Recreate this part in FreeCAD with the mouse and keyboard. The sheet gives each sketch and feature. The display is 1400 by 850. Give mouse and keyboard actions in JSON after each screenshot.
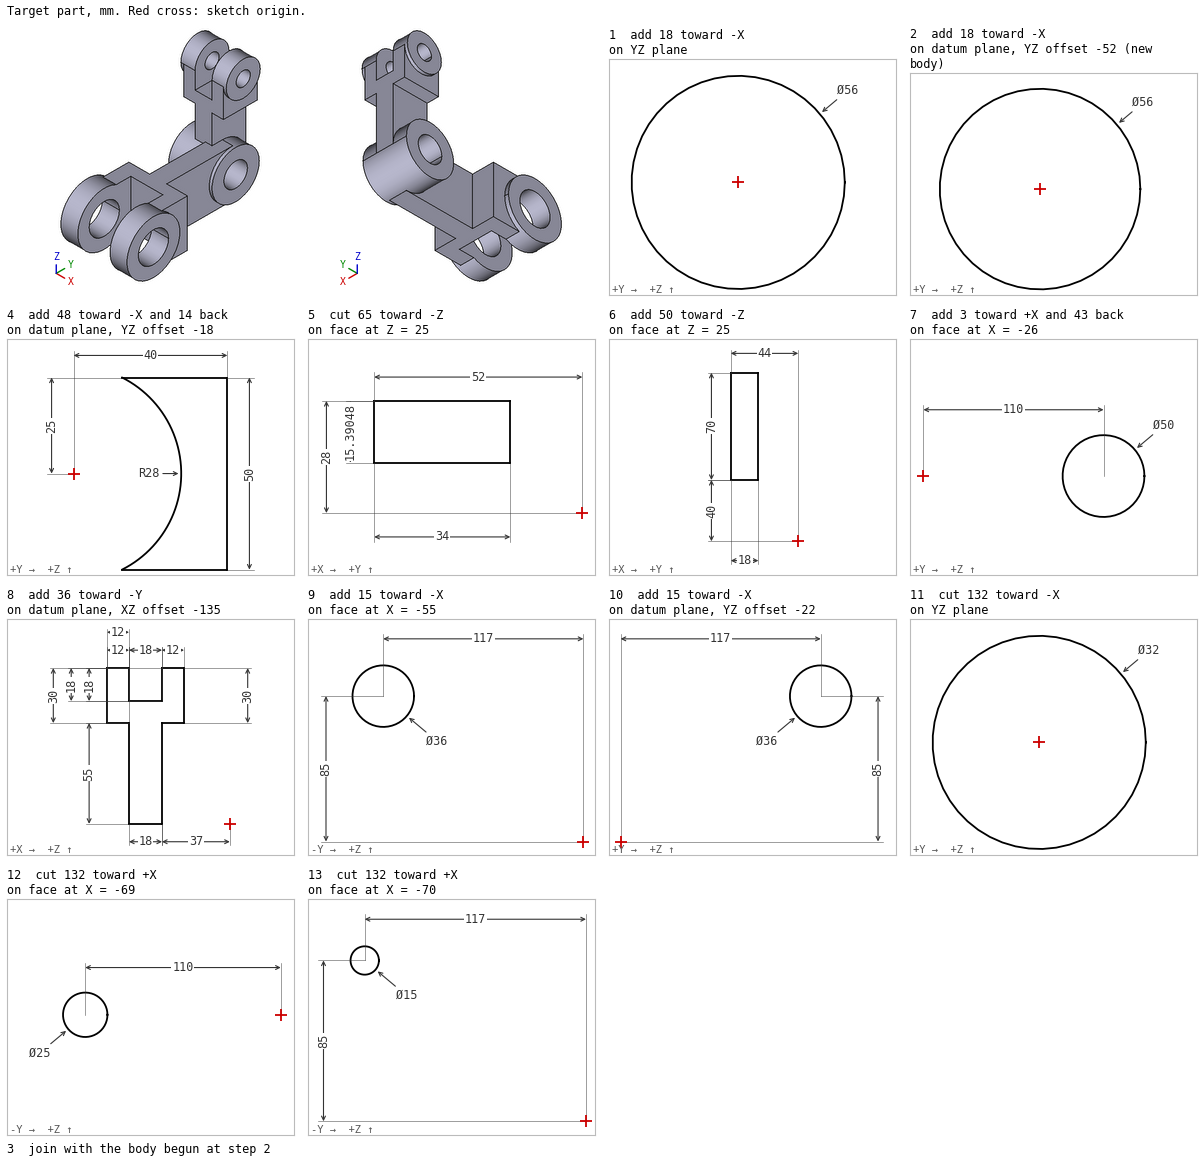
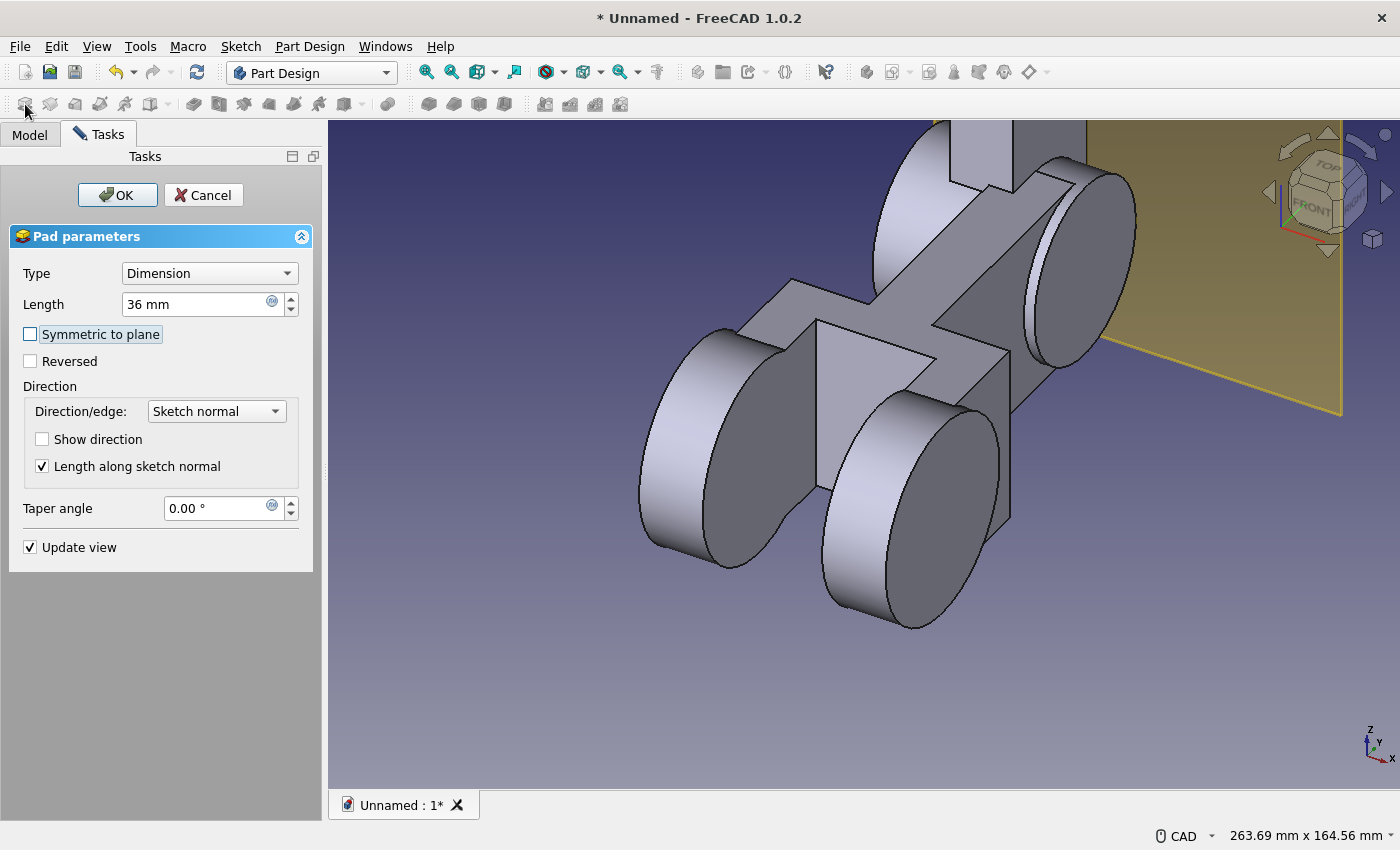
{"action": "left_click", "coordinate": [118, 195]}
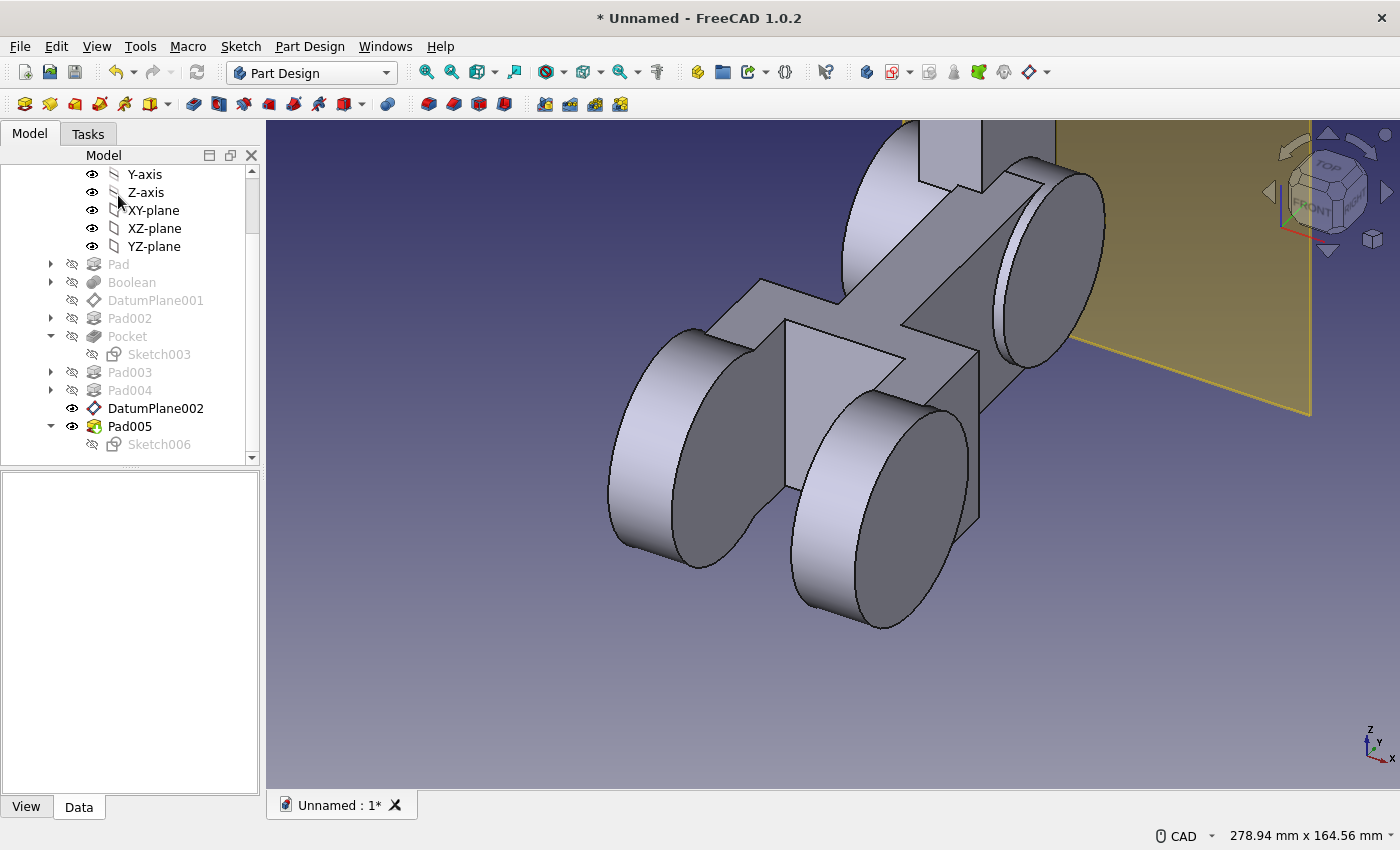
{"action": "left_click", "coordinate": [117, 408]}
{"action": "key", "text": "space"}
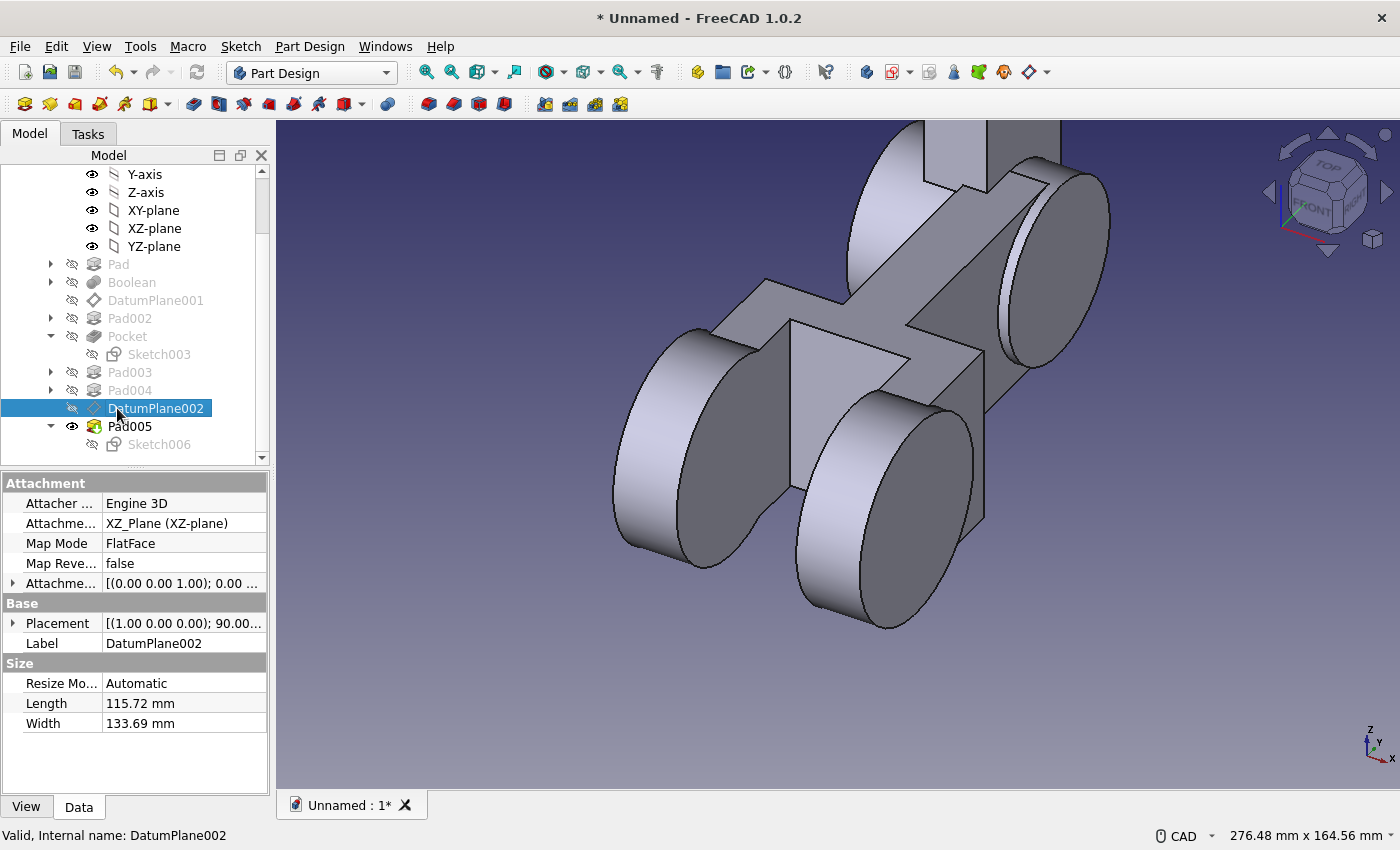
{"action": "left_click", "coordinate": [427, 72]}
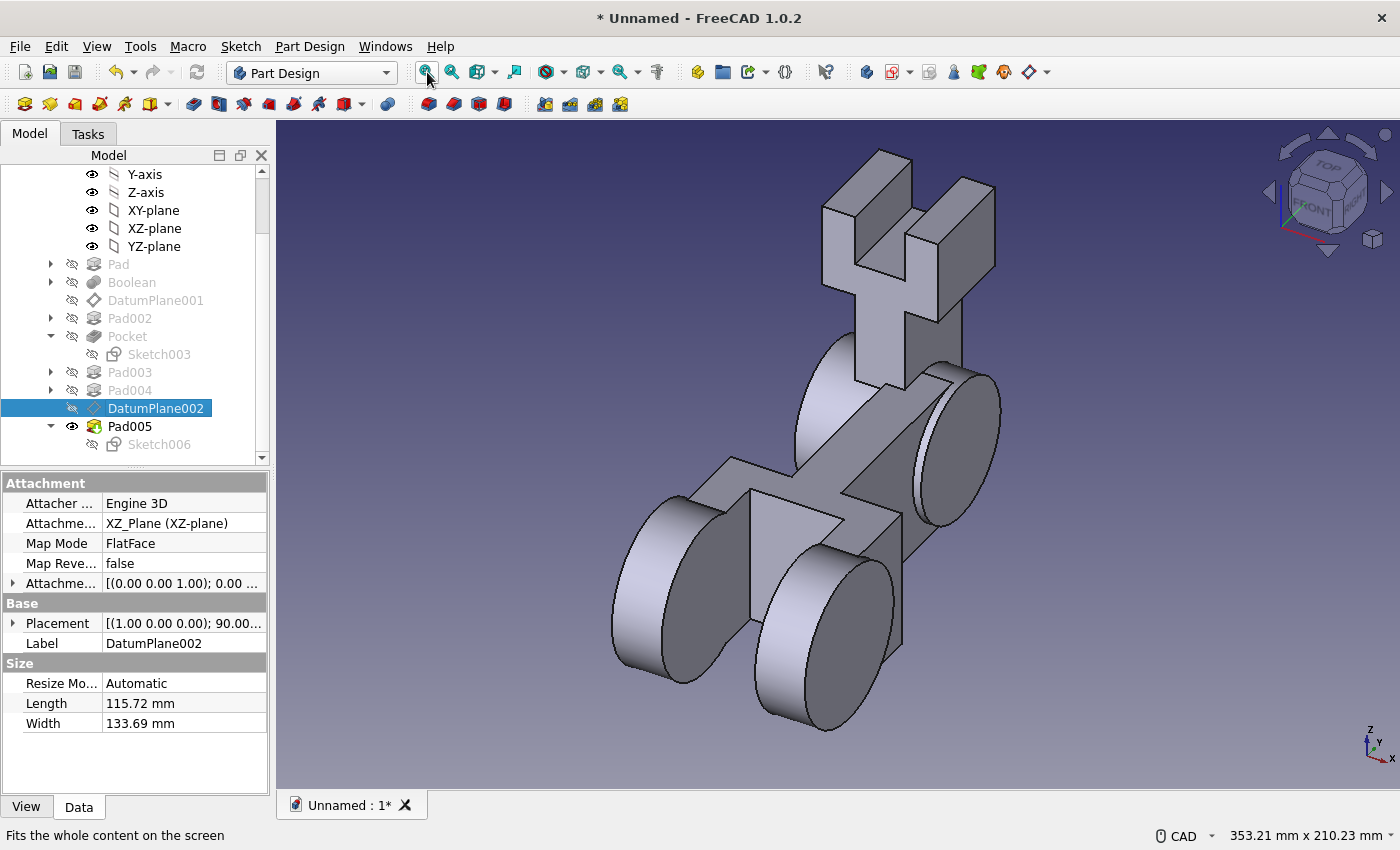
{"action": "key", "text": "6"}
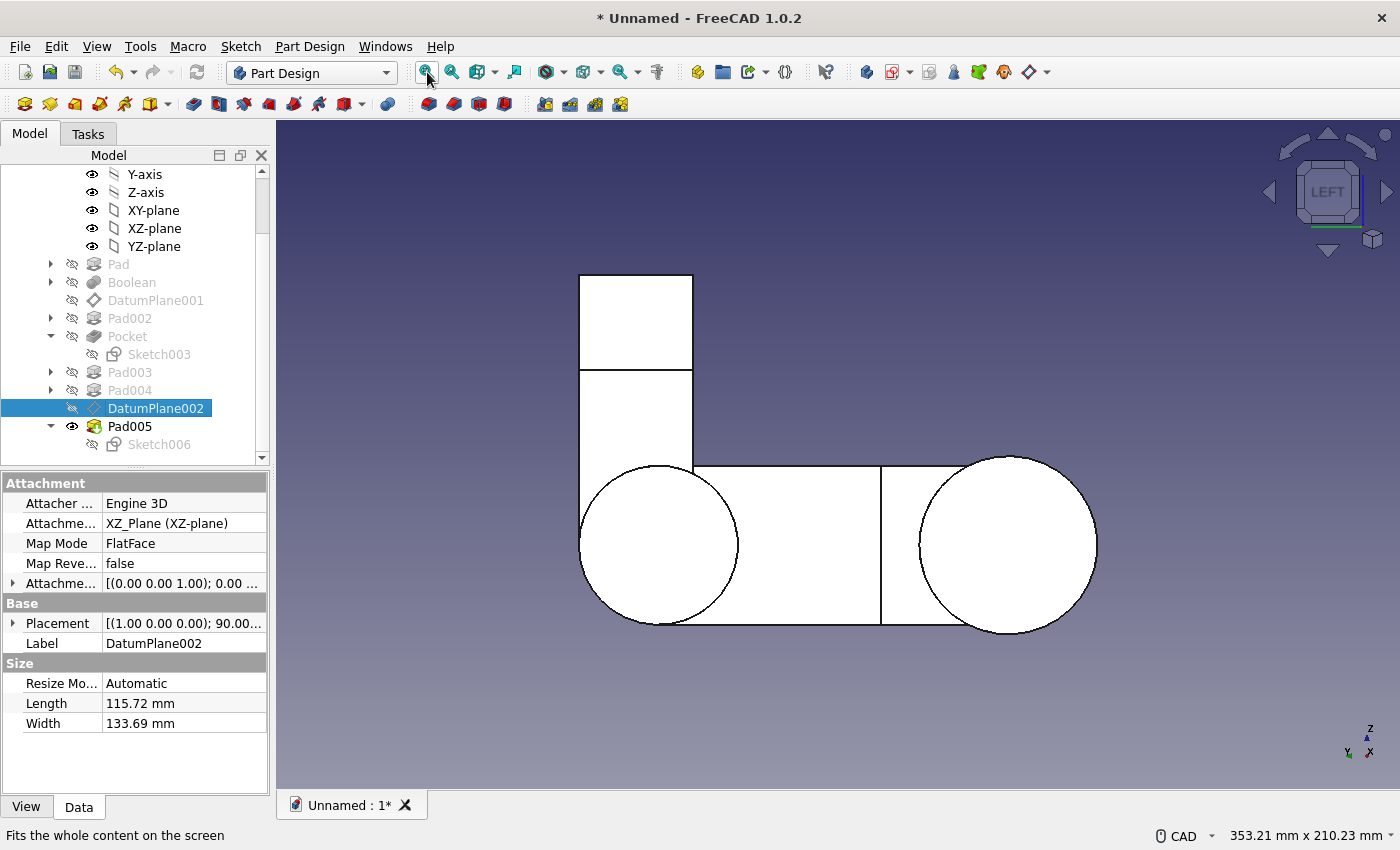
{"action": "left_click", "coordinate": [620, 432]}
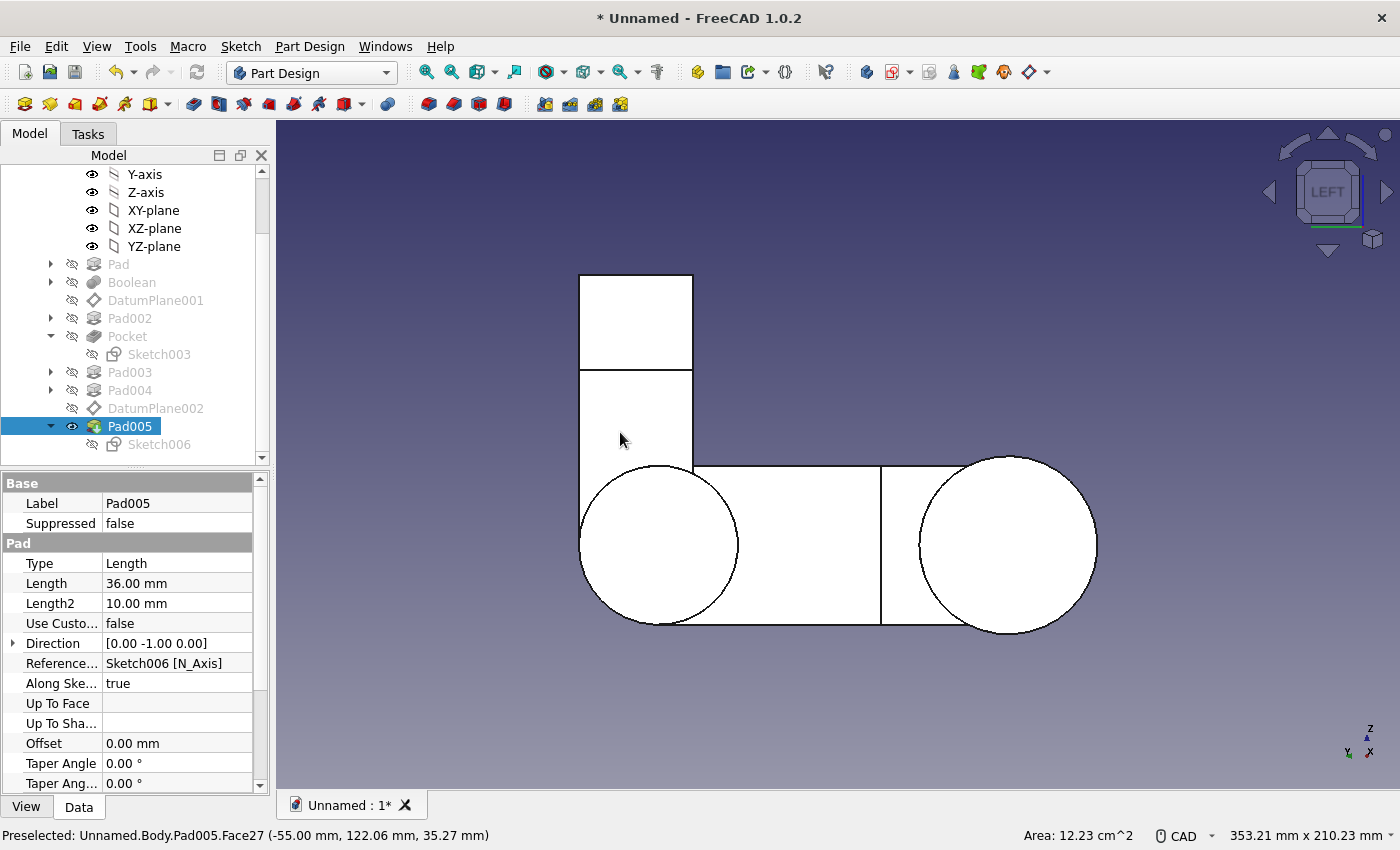
{"action": "left_click", "coordinate": [892, 72]}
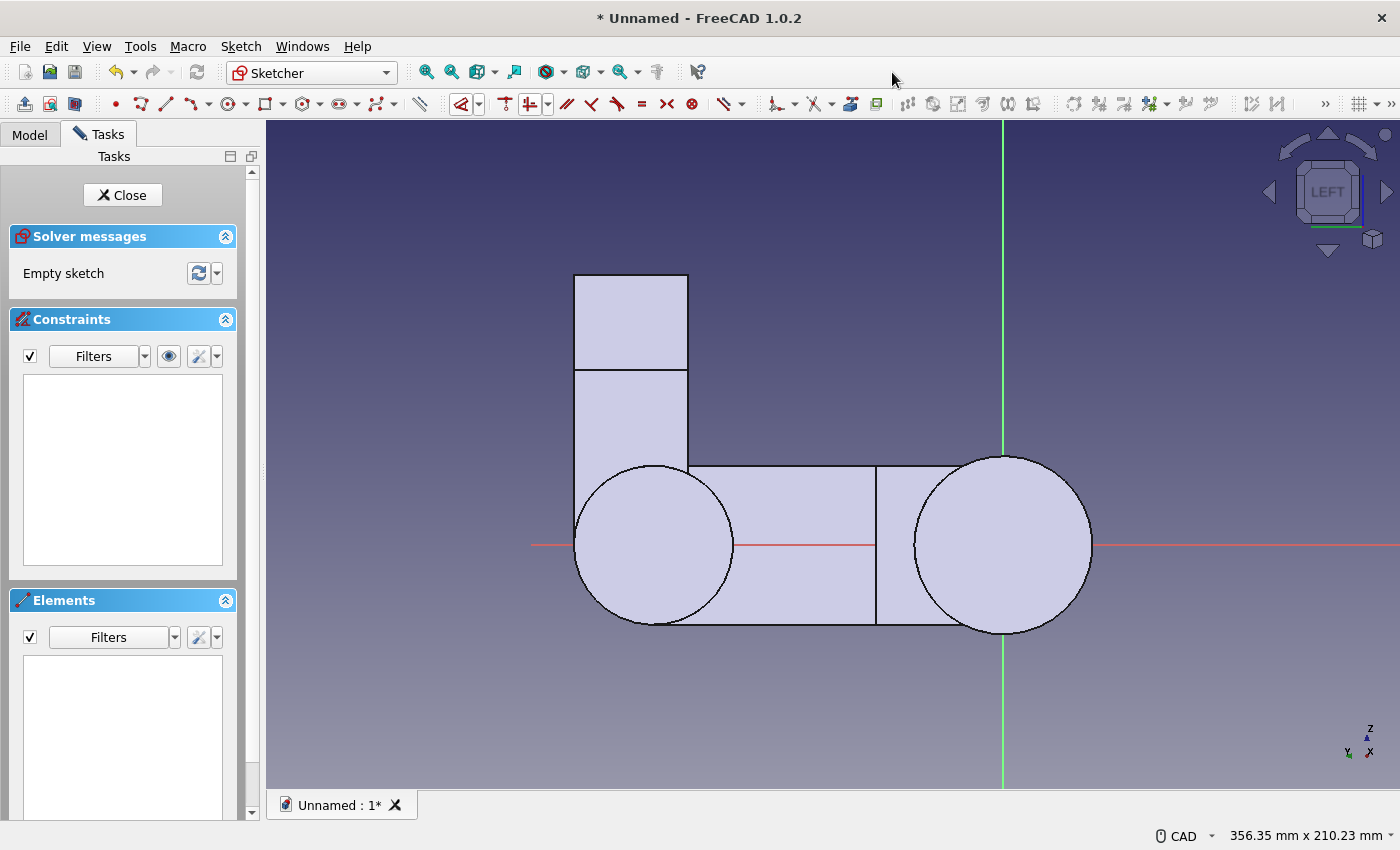
{"action": "scroll", "coordinate": [587, 216], "scroll_direction": "up", "scroll_amount": 7}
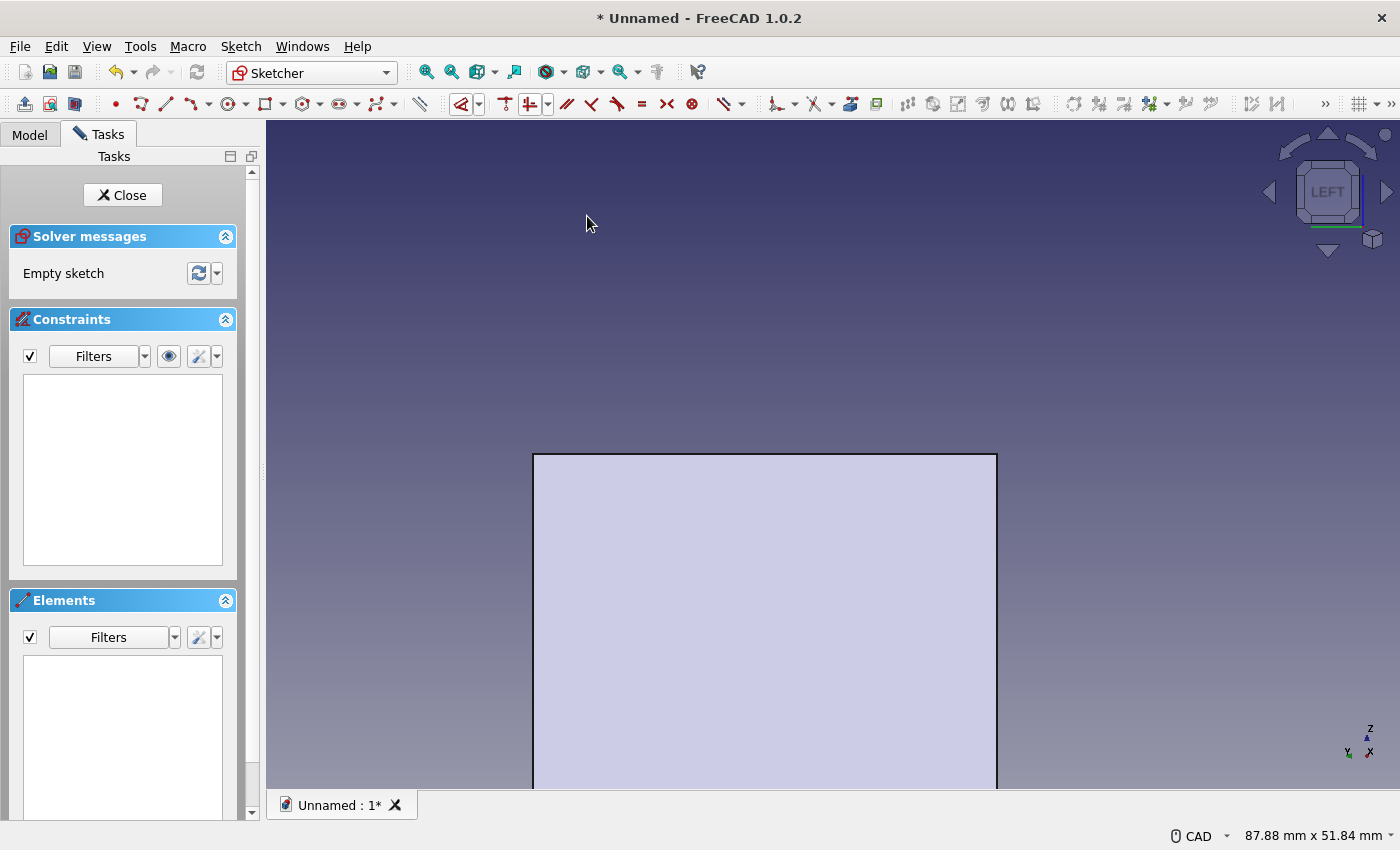
{"action": "key", "text": "g c"}